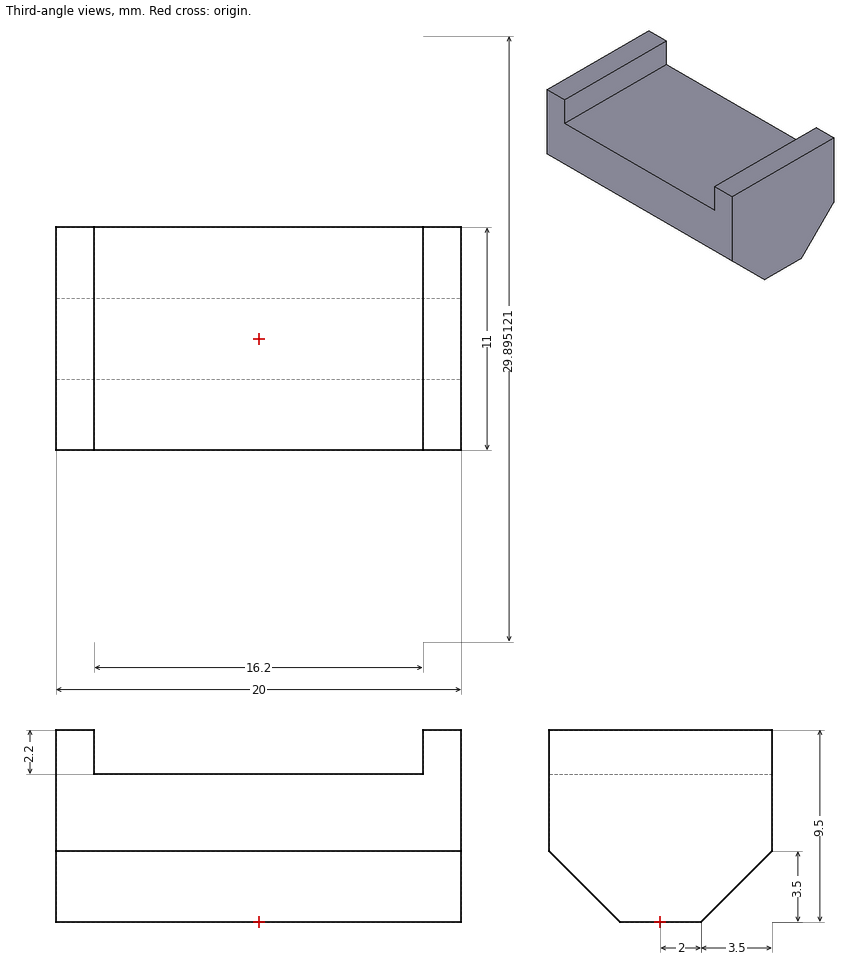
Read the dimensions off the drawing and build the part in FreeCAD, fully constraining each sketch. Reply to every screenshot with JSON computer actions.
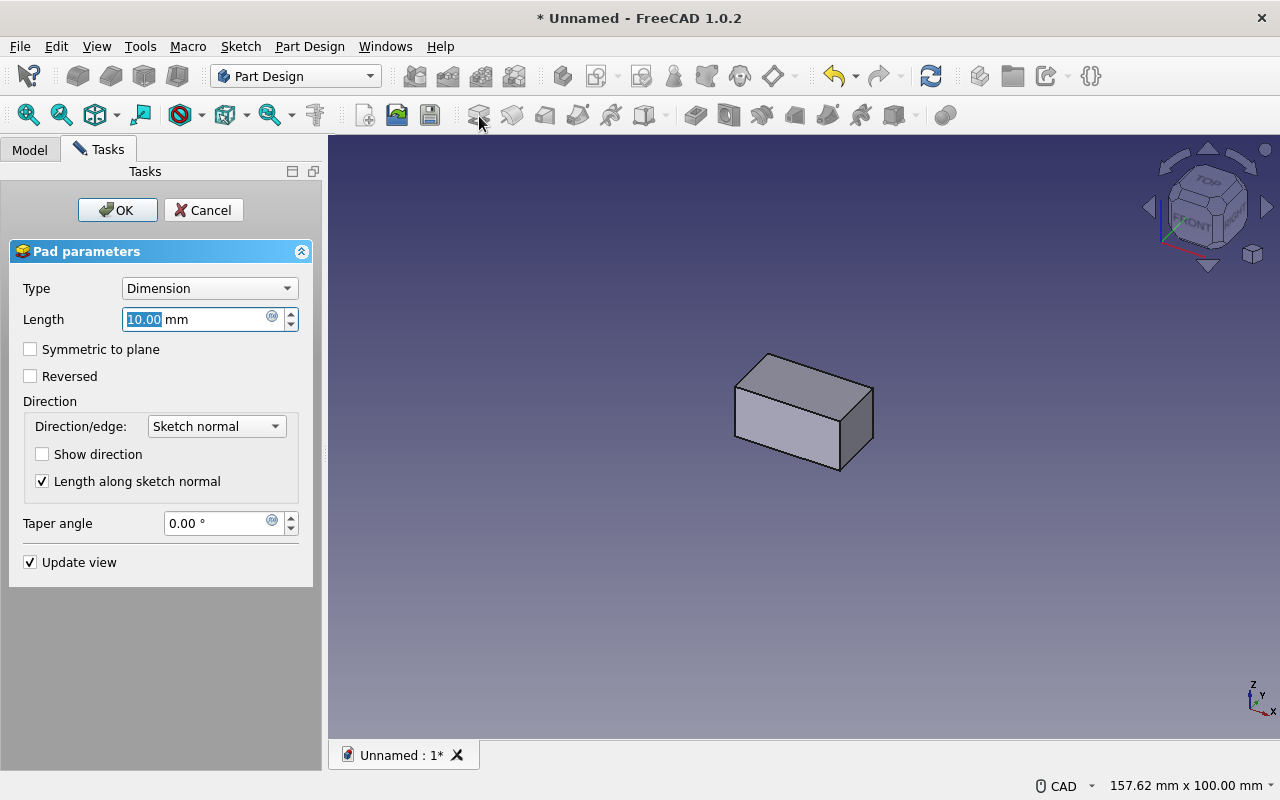
{"action": "type", "text": "9.5"}
{"action": "key", "text": "Tab"}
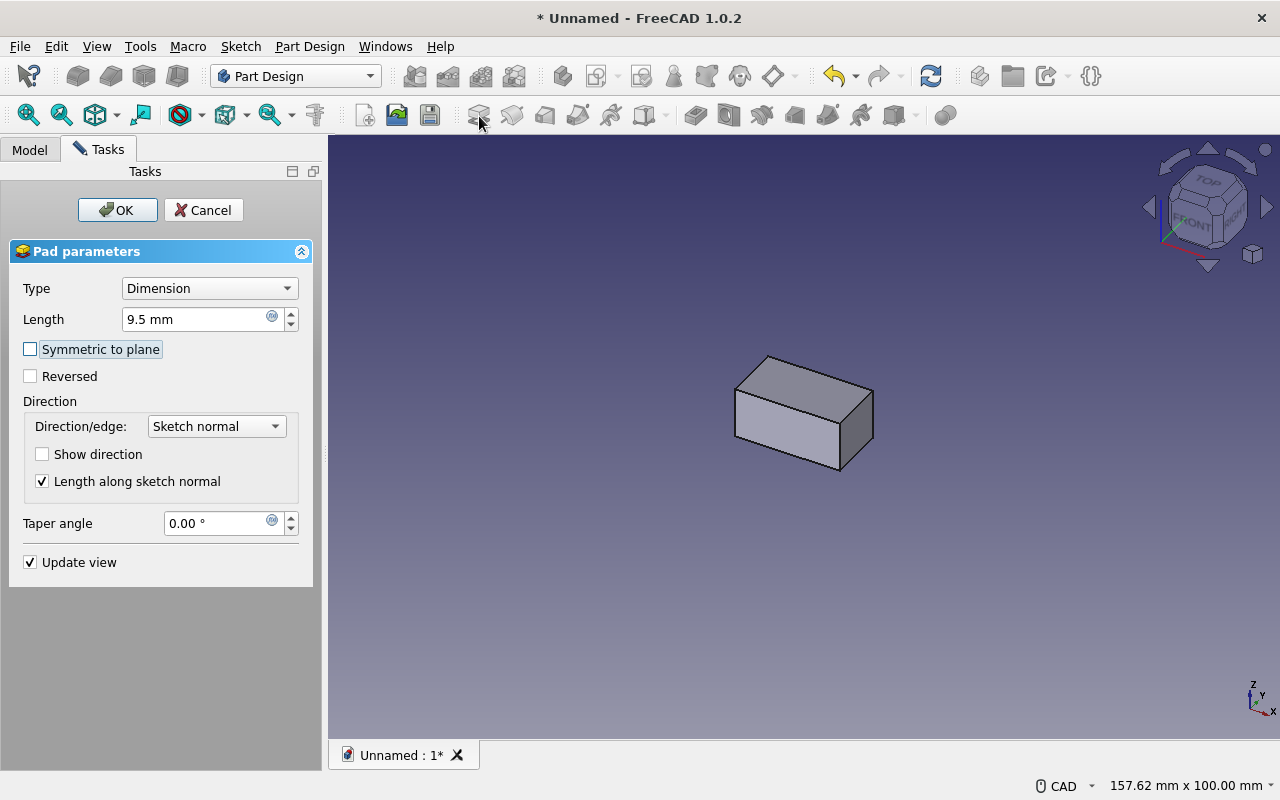
{"action": "left_click", "coordinate": [118, 210]}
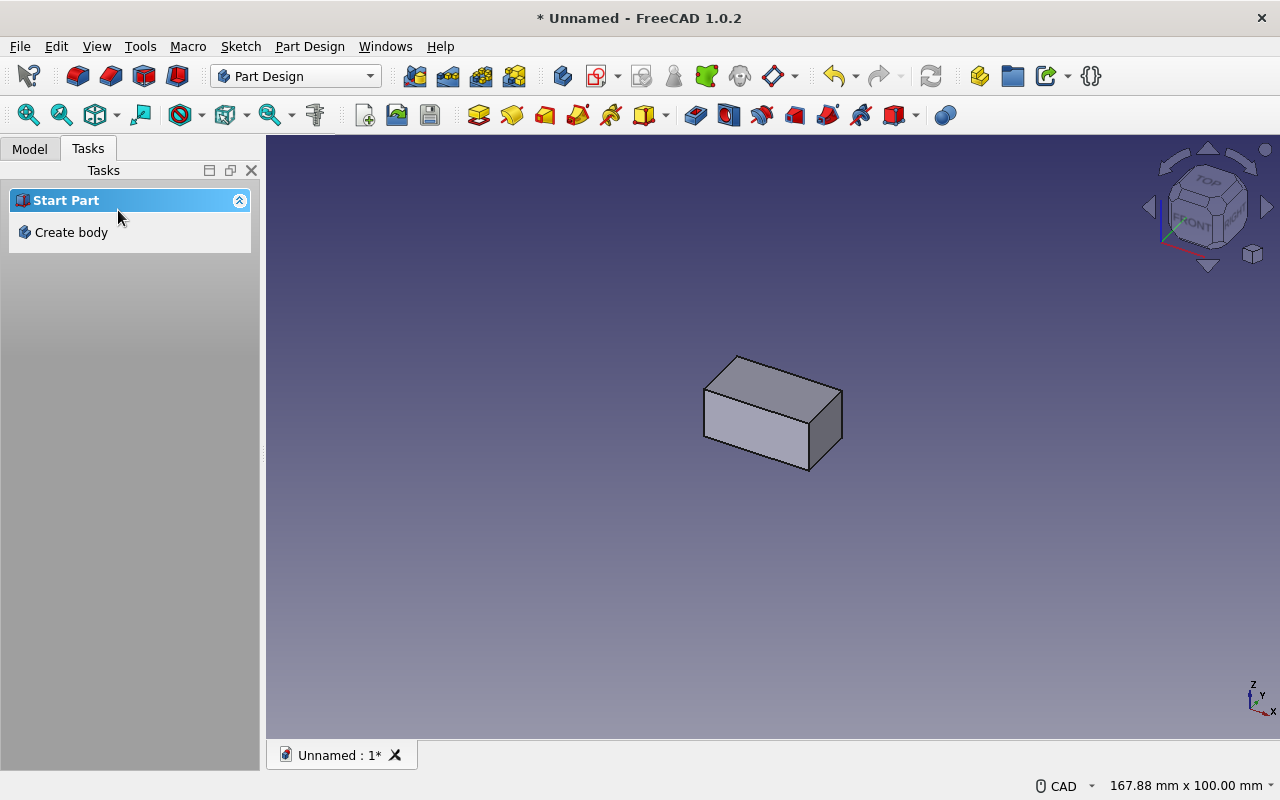
{"action": "left_click", "coordinate": [29, 116]}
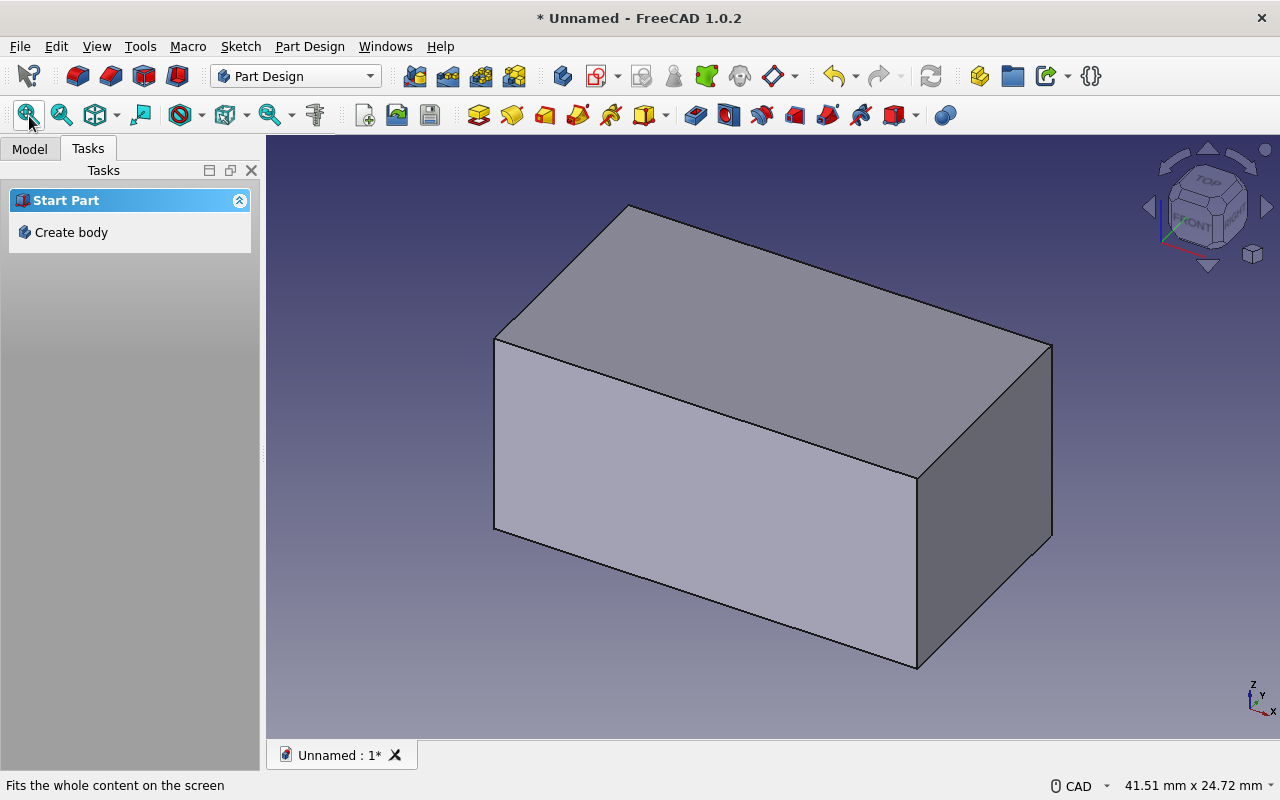
{"action": "left_click", "coordinate": [833, 361]}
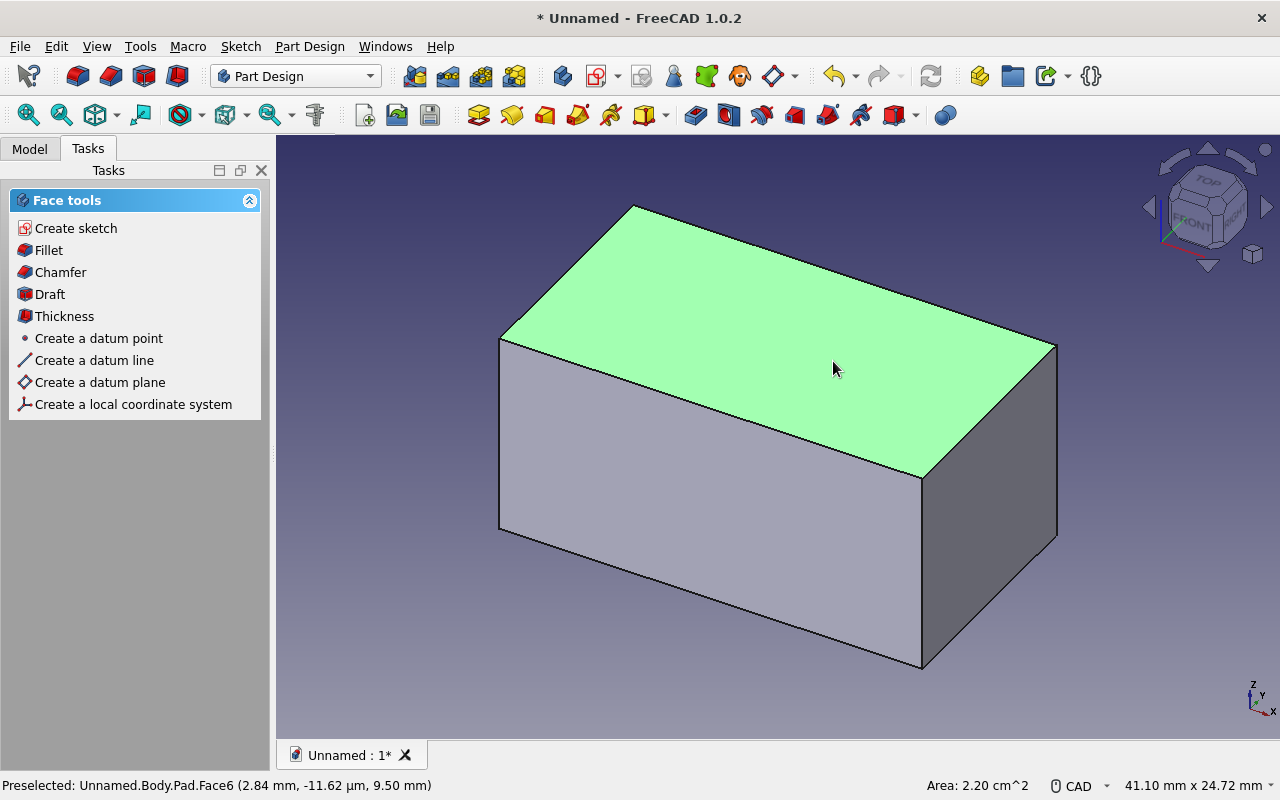
{"action": "left_click", "coordinate": [596, 76]}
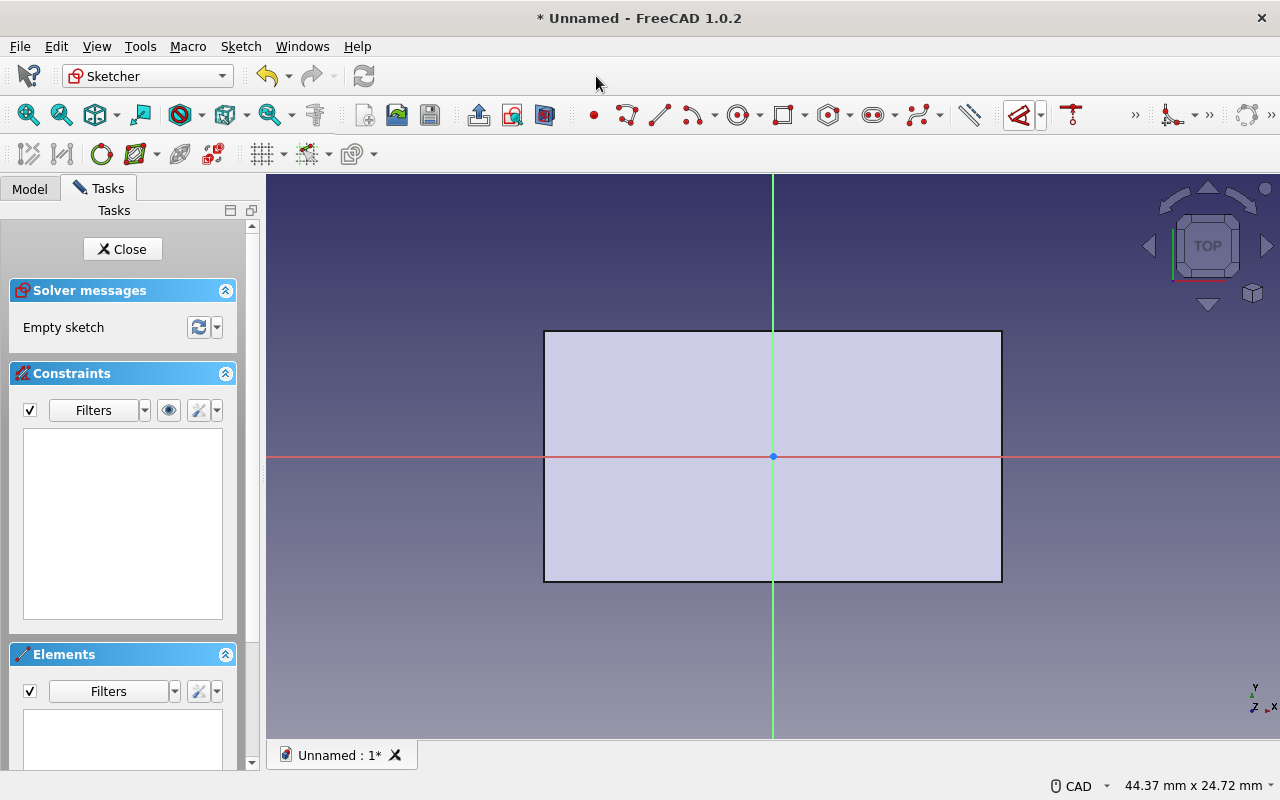
{"action": "scroll", "coordinate": [621, 456], "scroll_direction": "down", "scroll_amount": 3}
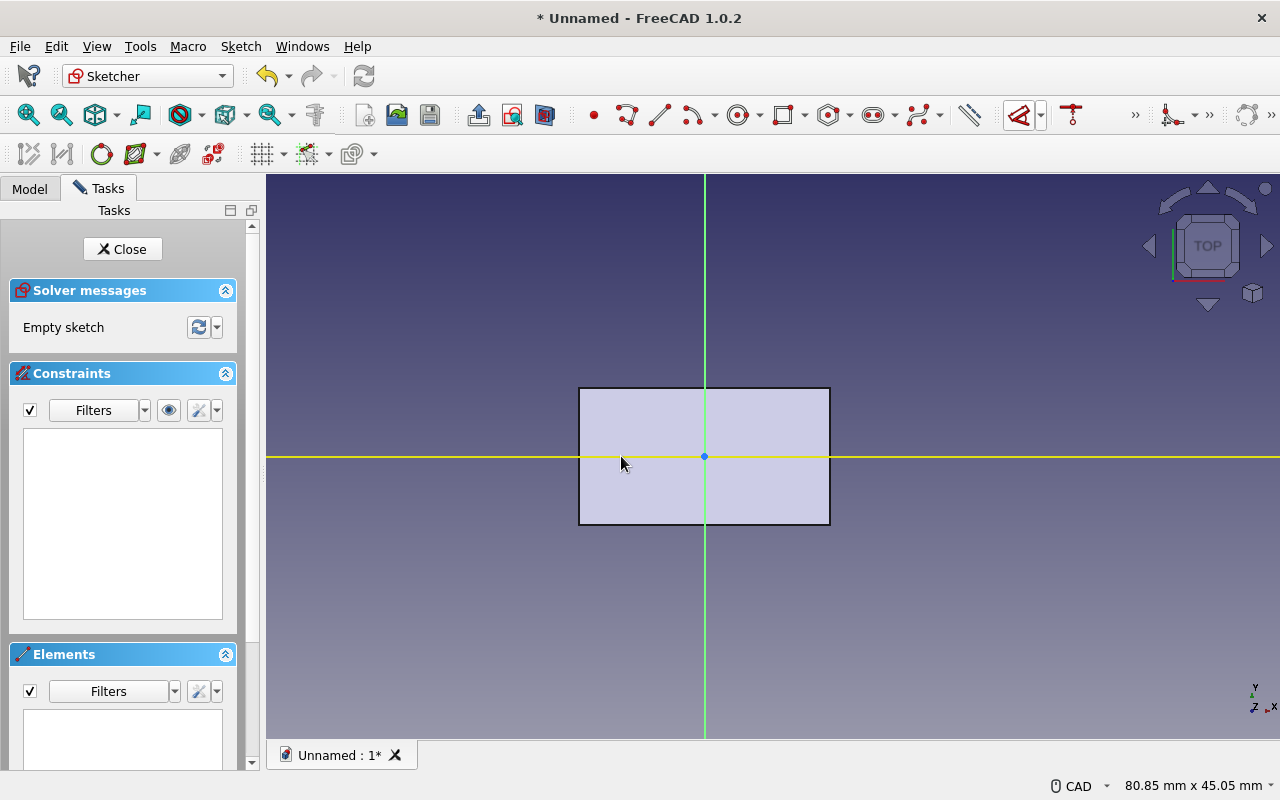
{"action": "left_click", "coordinate": [804, 116]}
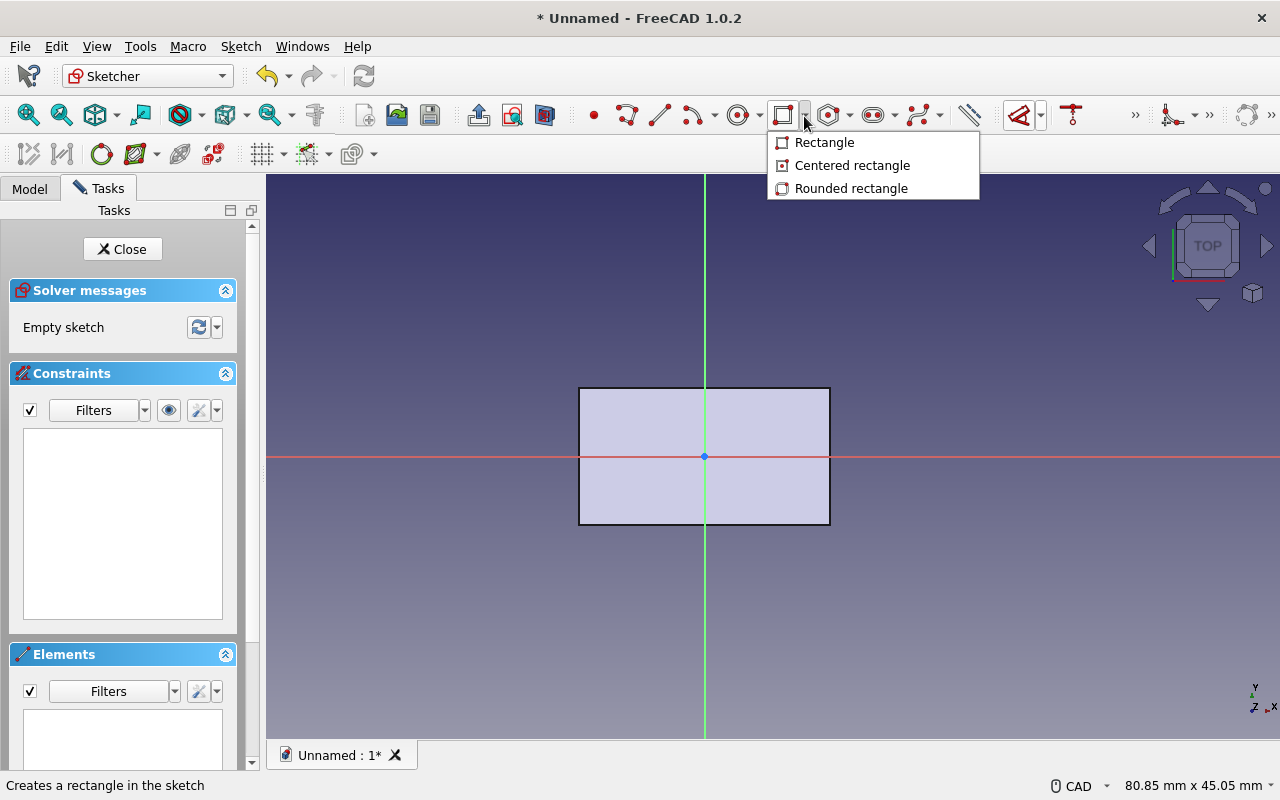
{"action": "left_click", "coordinate": [874, 166]}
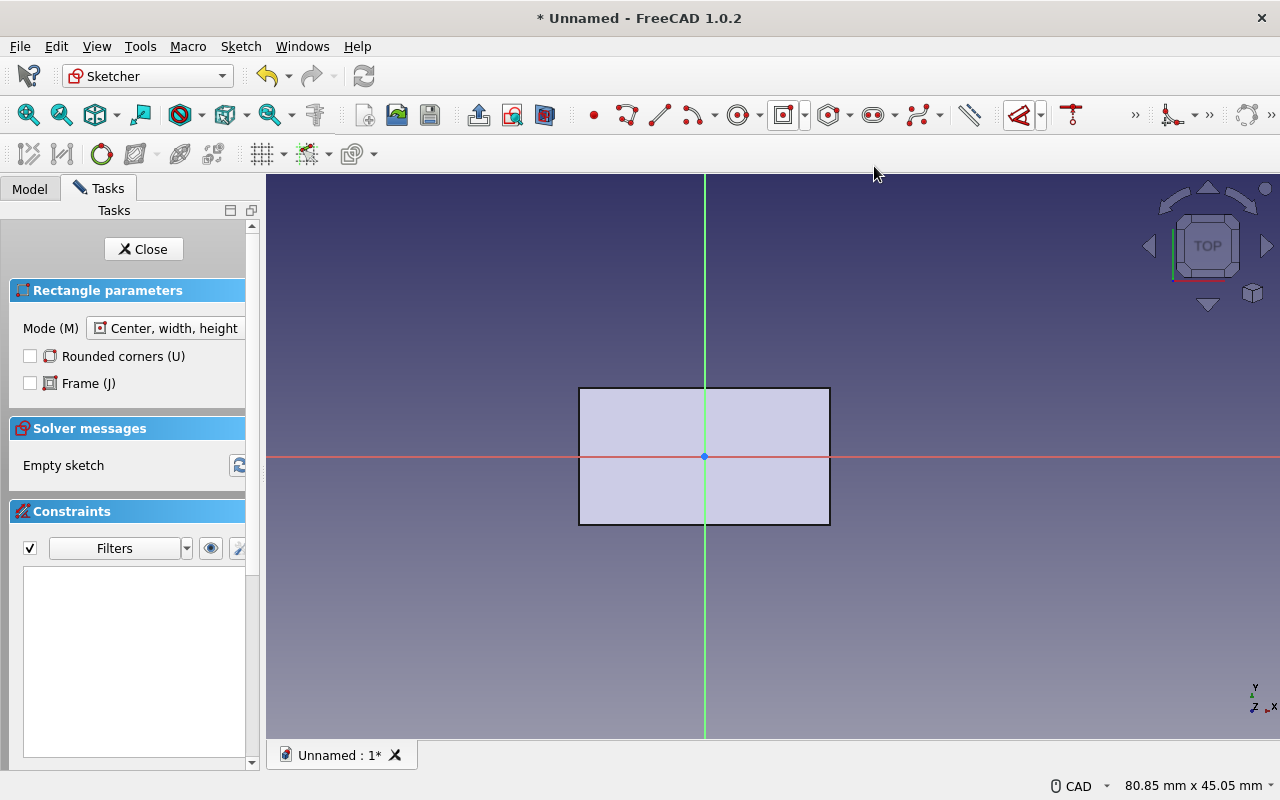
{"action": "left_click", "coordinate": [705, 456]}
{"action": "mouse_move", "coordinate": [806, 269]}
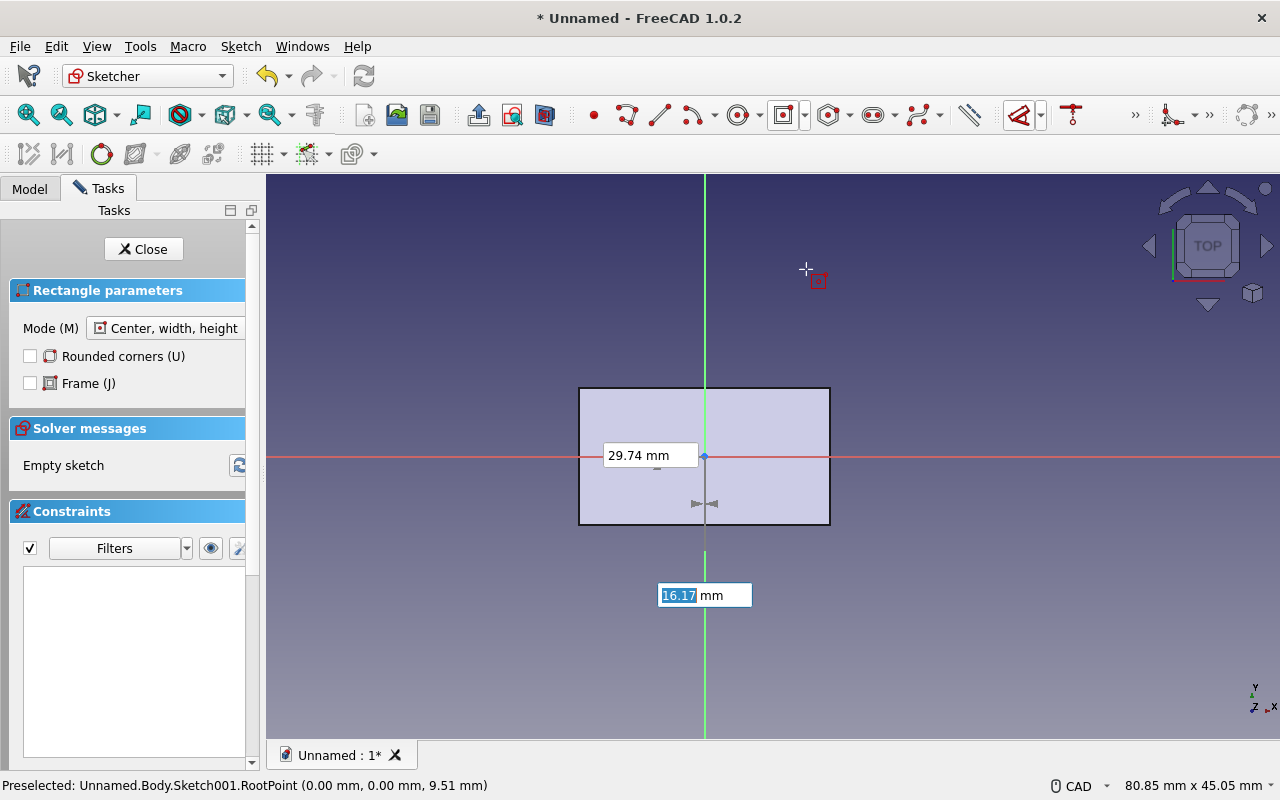
{"action": "type", "text": "16.2"}
{"action": "key", "text": "Tab"}
{"action": "type", "text": "29.895121"}
{"action": "key", "text": "Return"}
{"action": "key", "text": "Escape"}